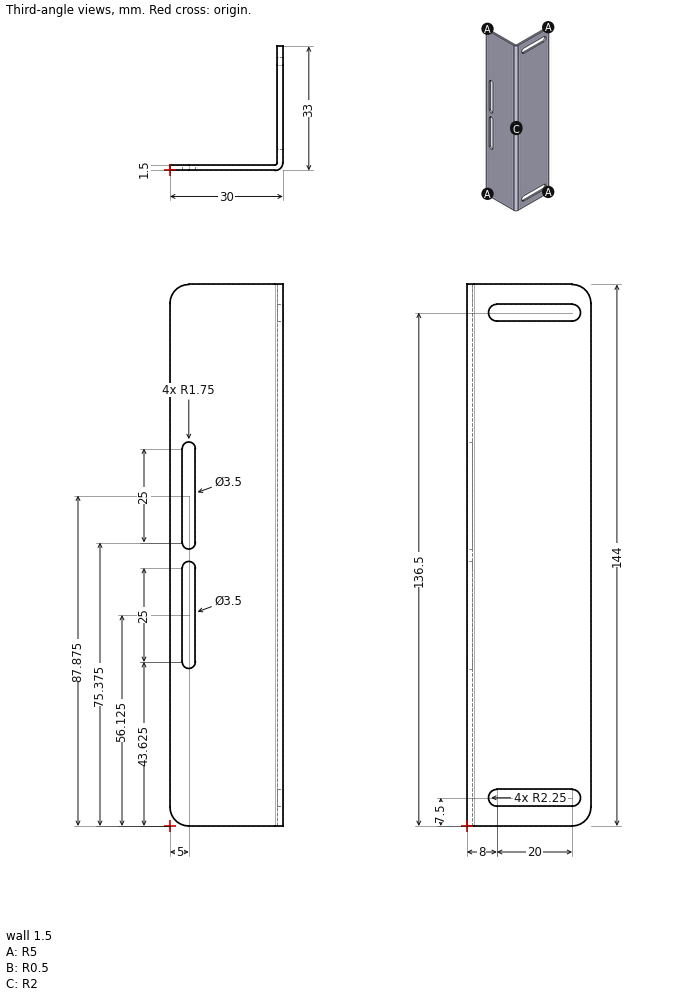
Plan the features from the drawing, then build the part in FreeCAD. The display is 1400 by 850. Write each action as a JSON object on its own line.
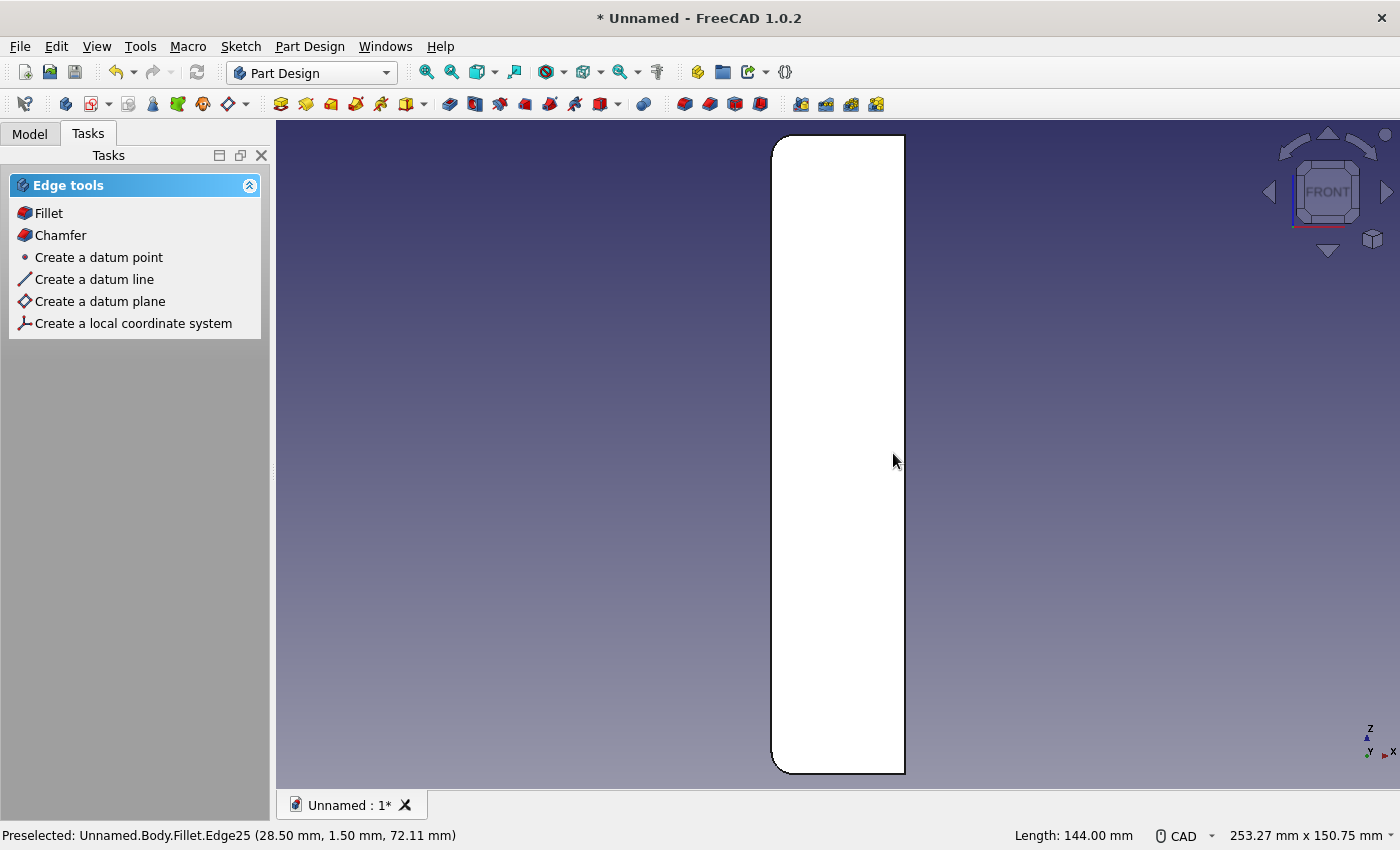
{"action": "left_click", "coordinate": [685, 104]}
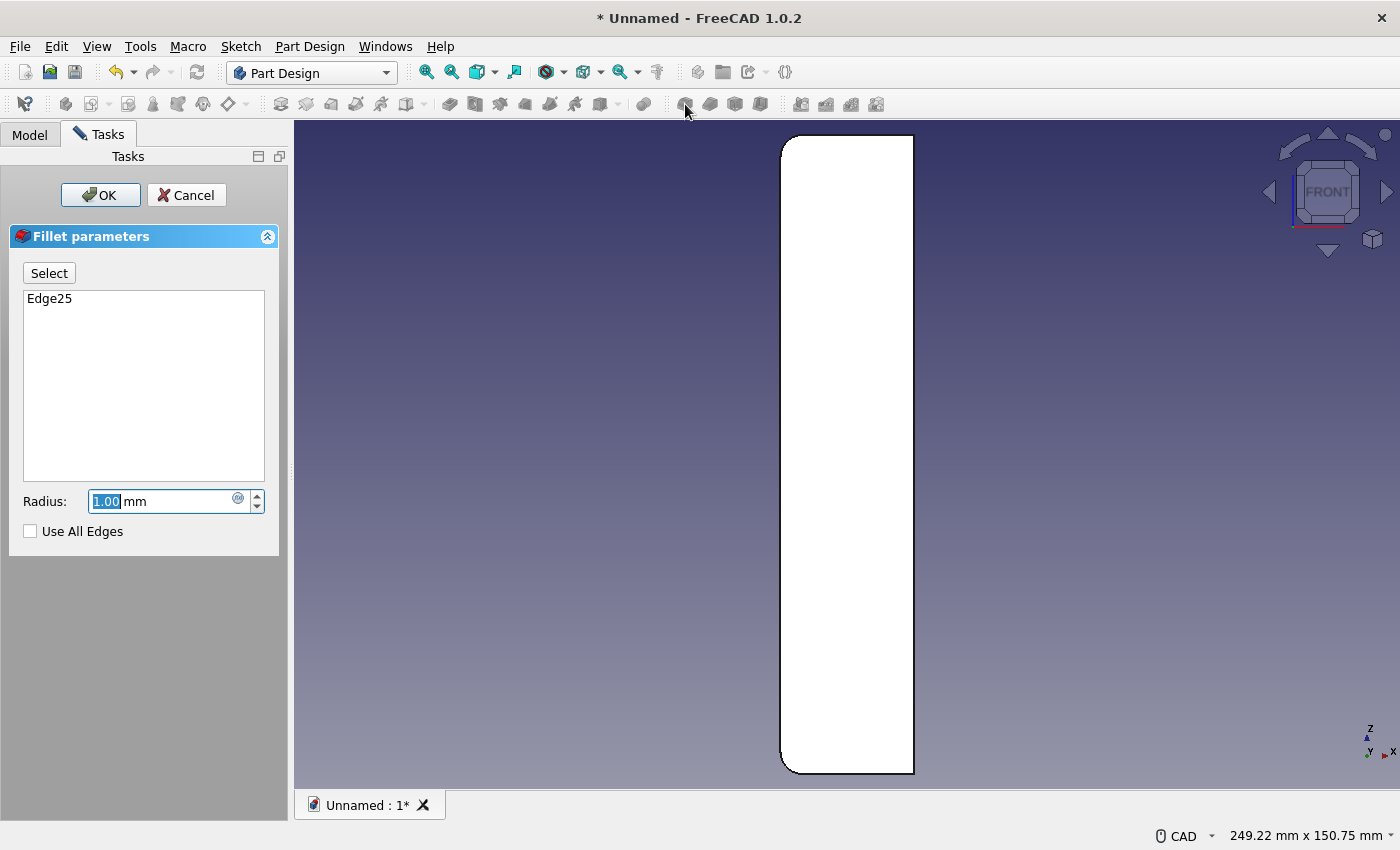
{"action": "type", "text": "0.5"}
{"action": "key", "text": "Tab"}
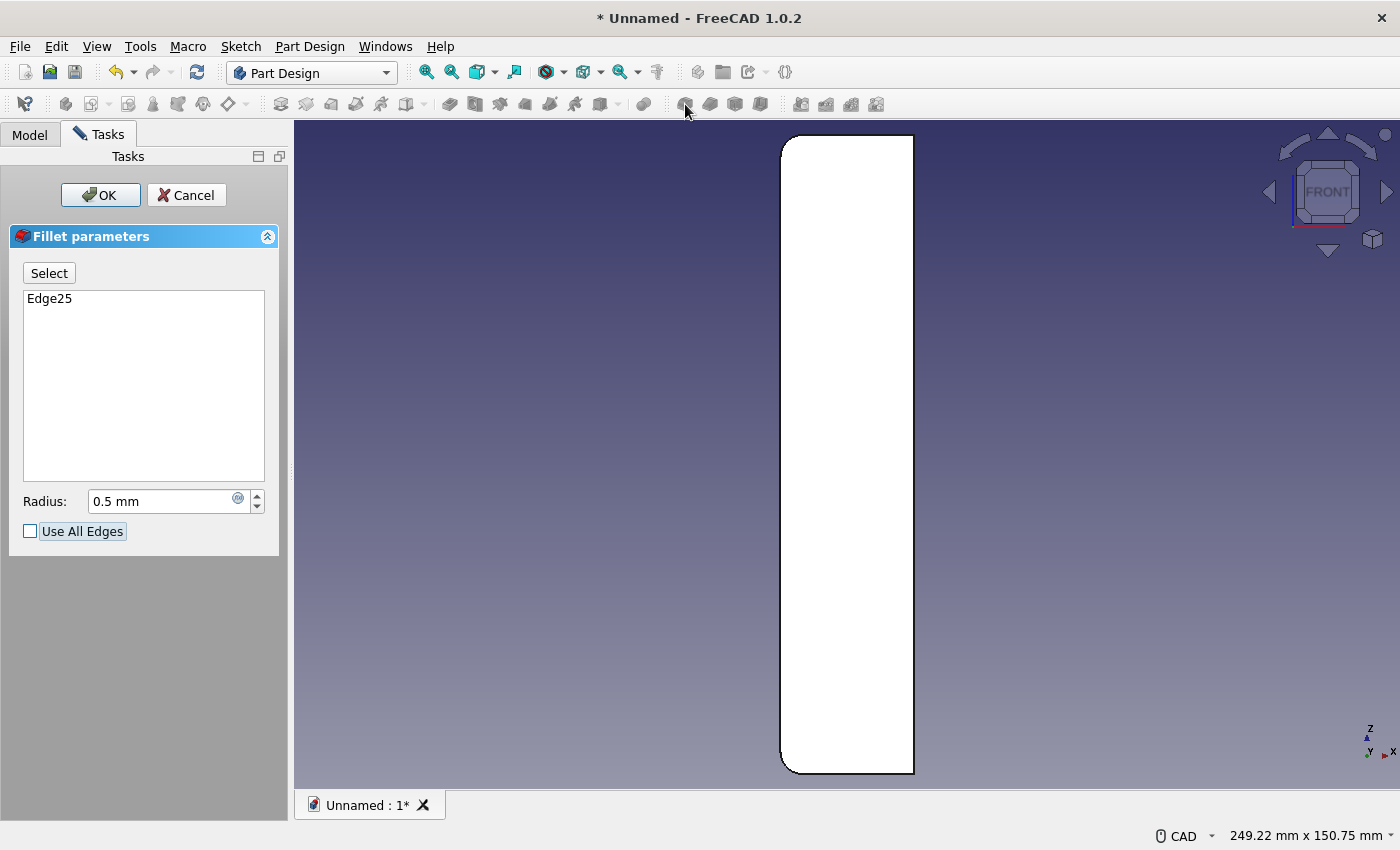
{"action": "left_click", "coordinate": [101, 195]}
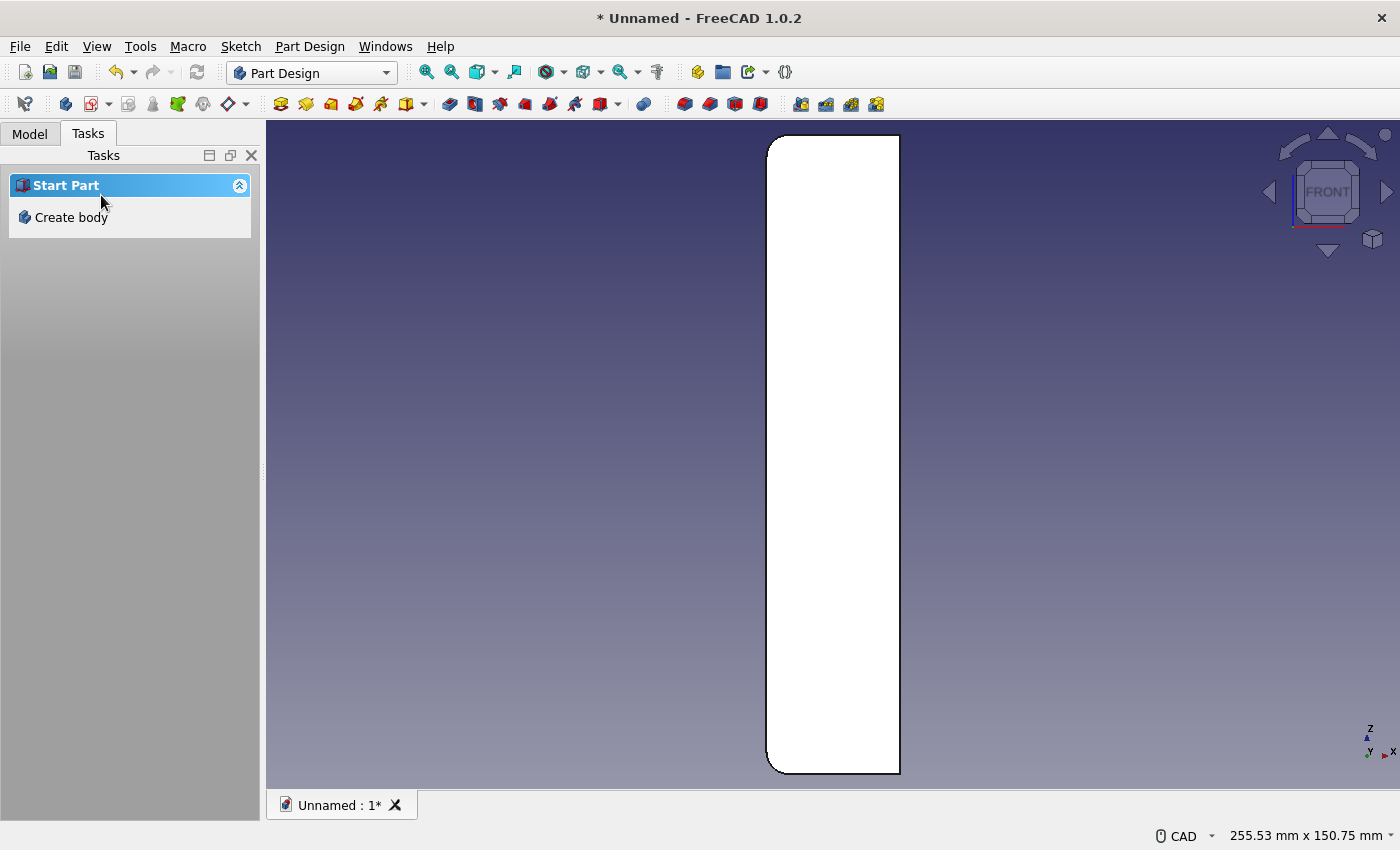
{"action": "left_click", "coordinate": [900, 453]}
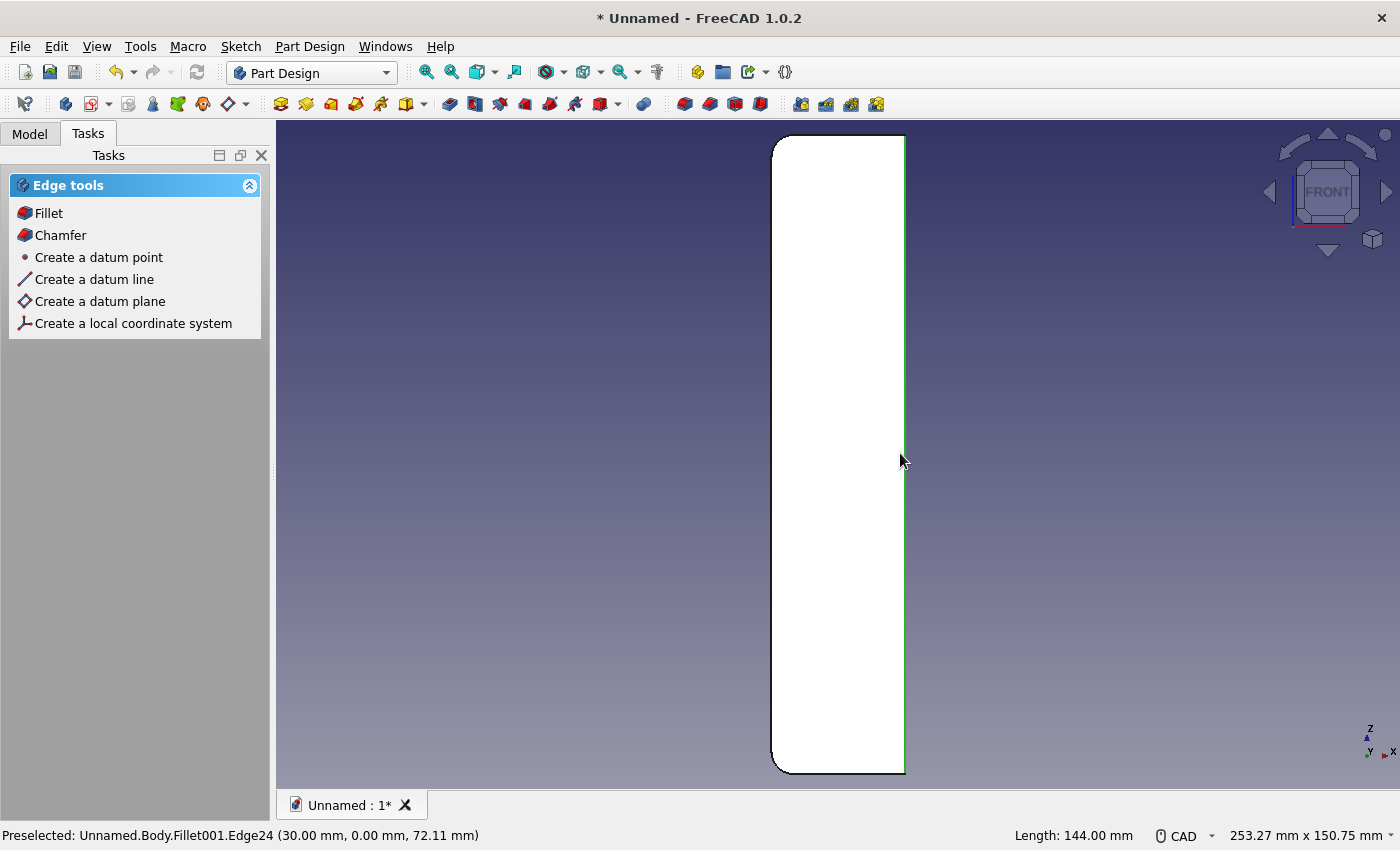
{"action": "left_click", "coordinate": [685, 104]}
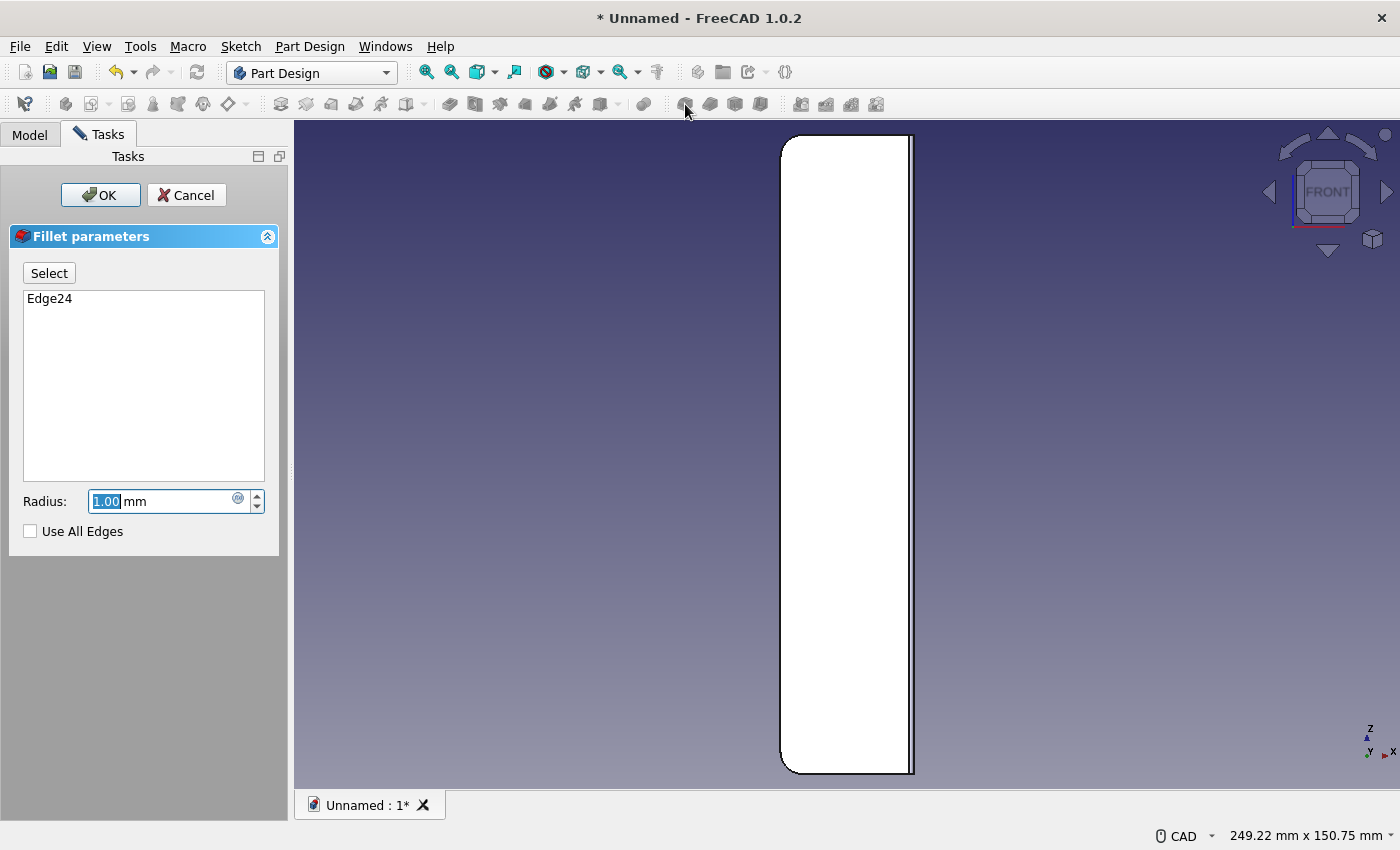
{"action": "type", "text": "2"}
{"action": "key", "text": "Tab"}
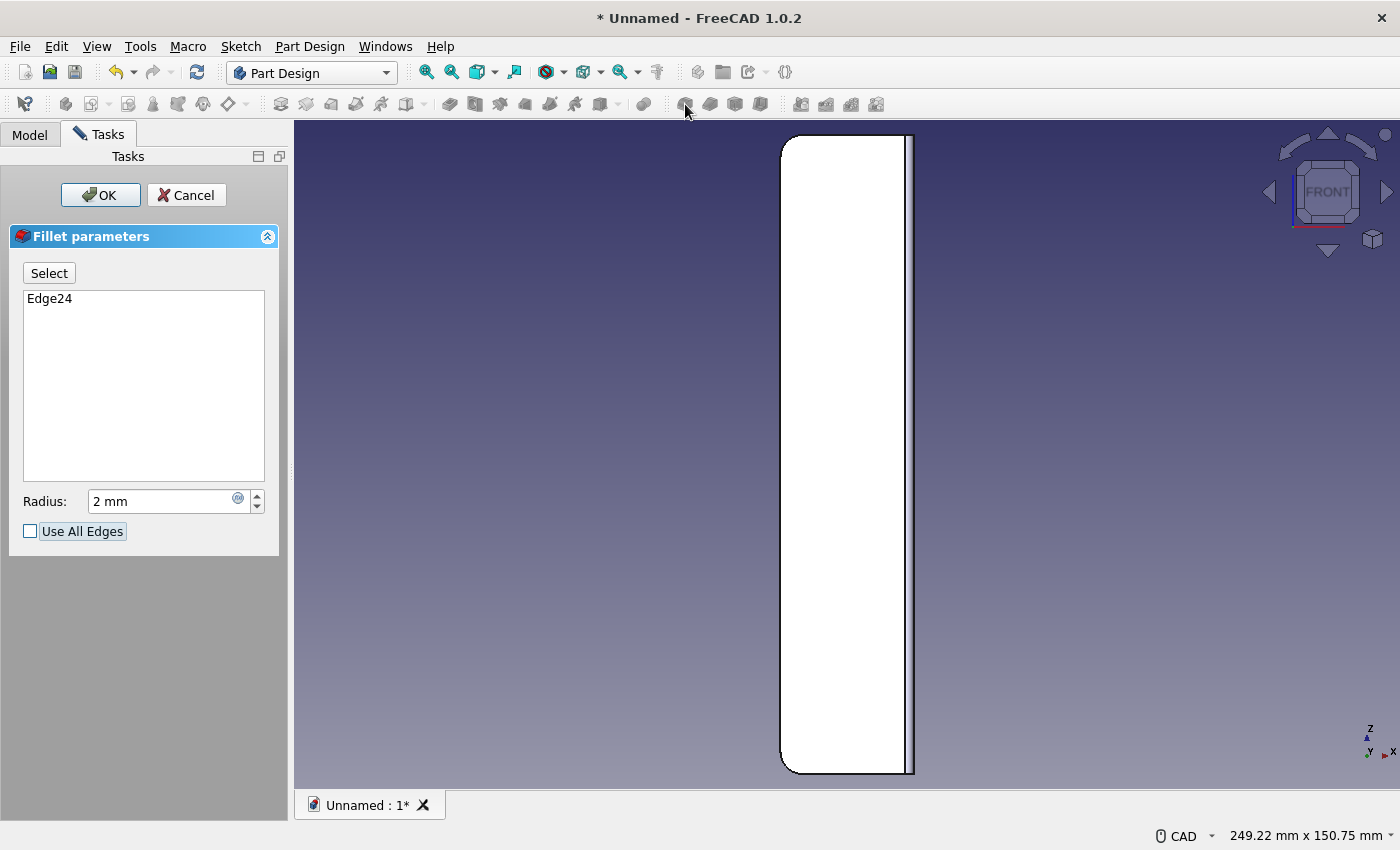
{"action": "left_click", "coordinate": [101, 195]}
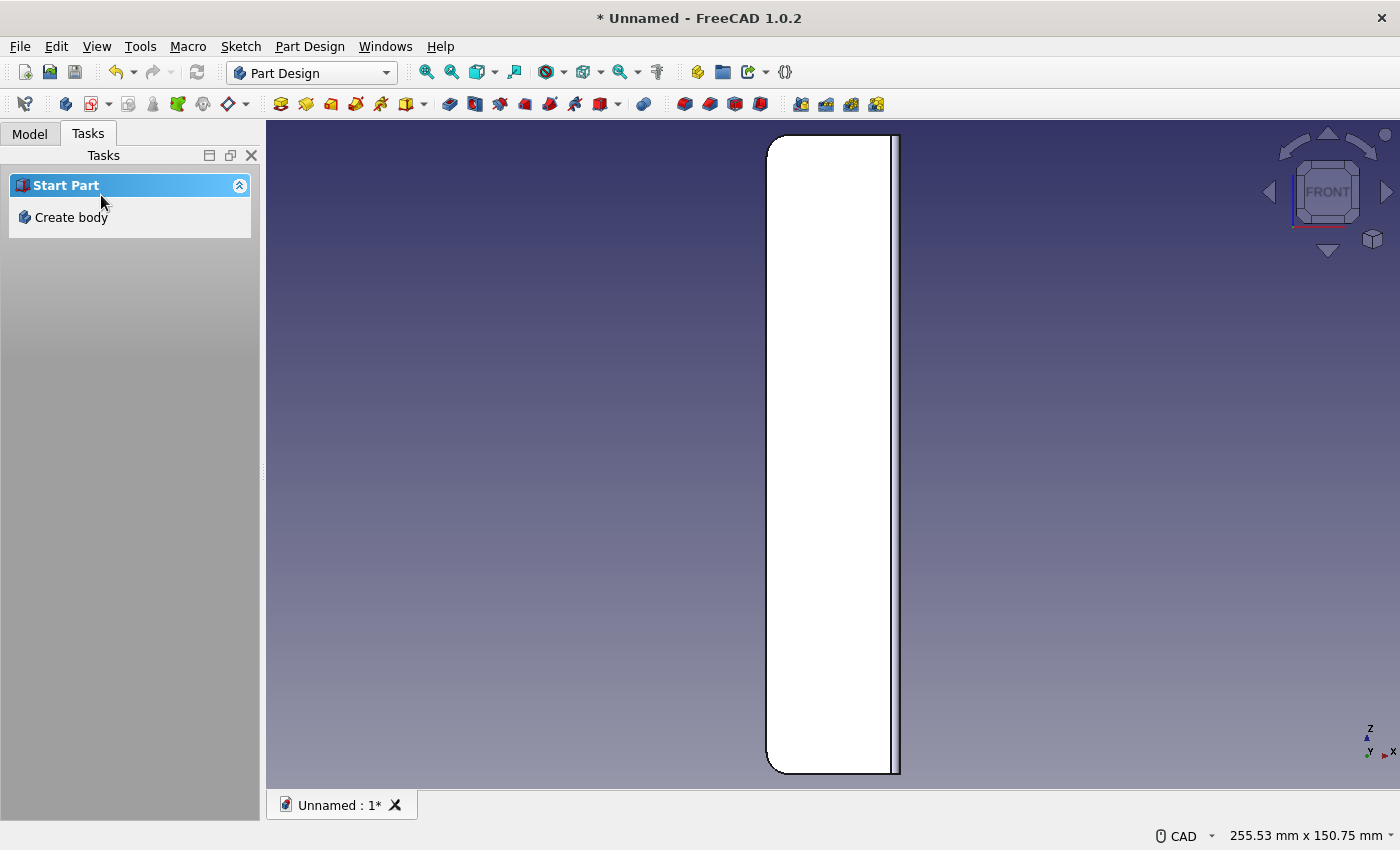
{"action": "key", "text": "6"}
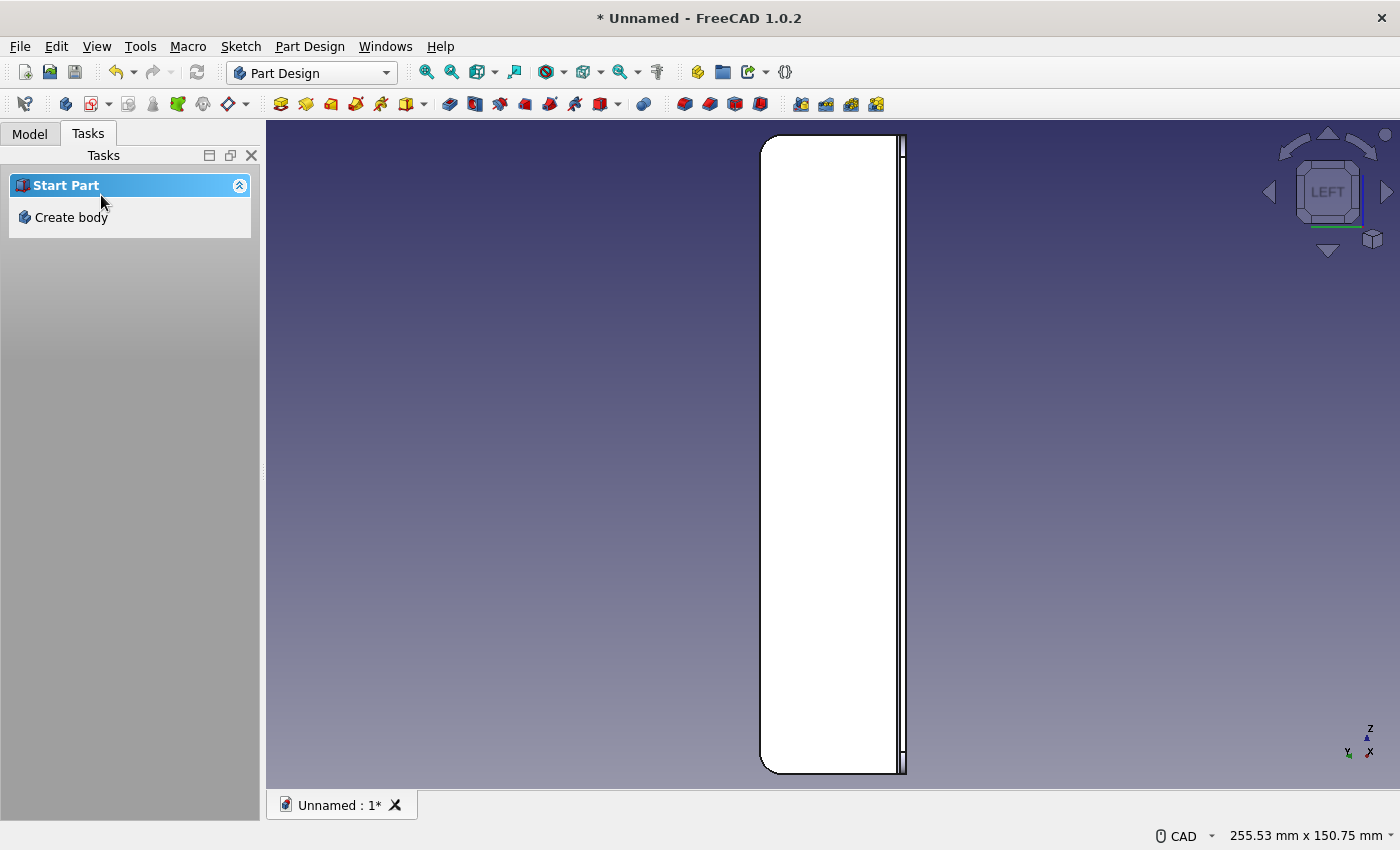
{"action": "left_click", "coordinate": [829, 271]}